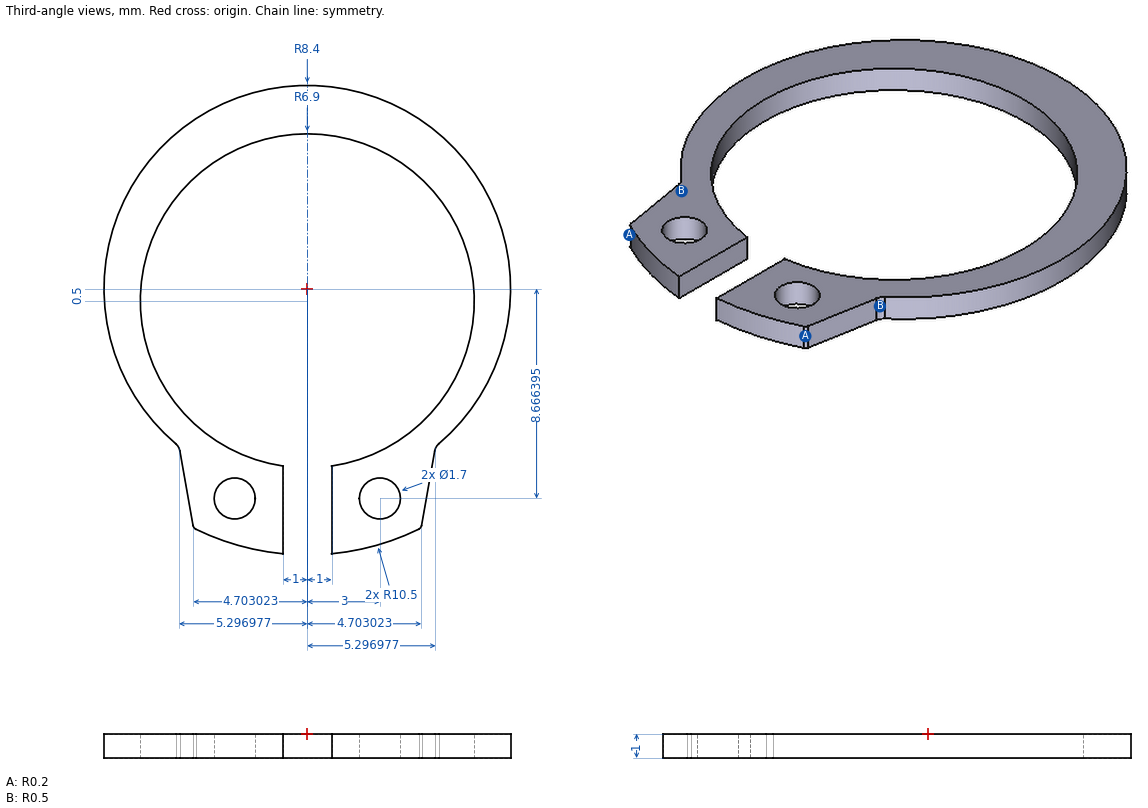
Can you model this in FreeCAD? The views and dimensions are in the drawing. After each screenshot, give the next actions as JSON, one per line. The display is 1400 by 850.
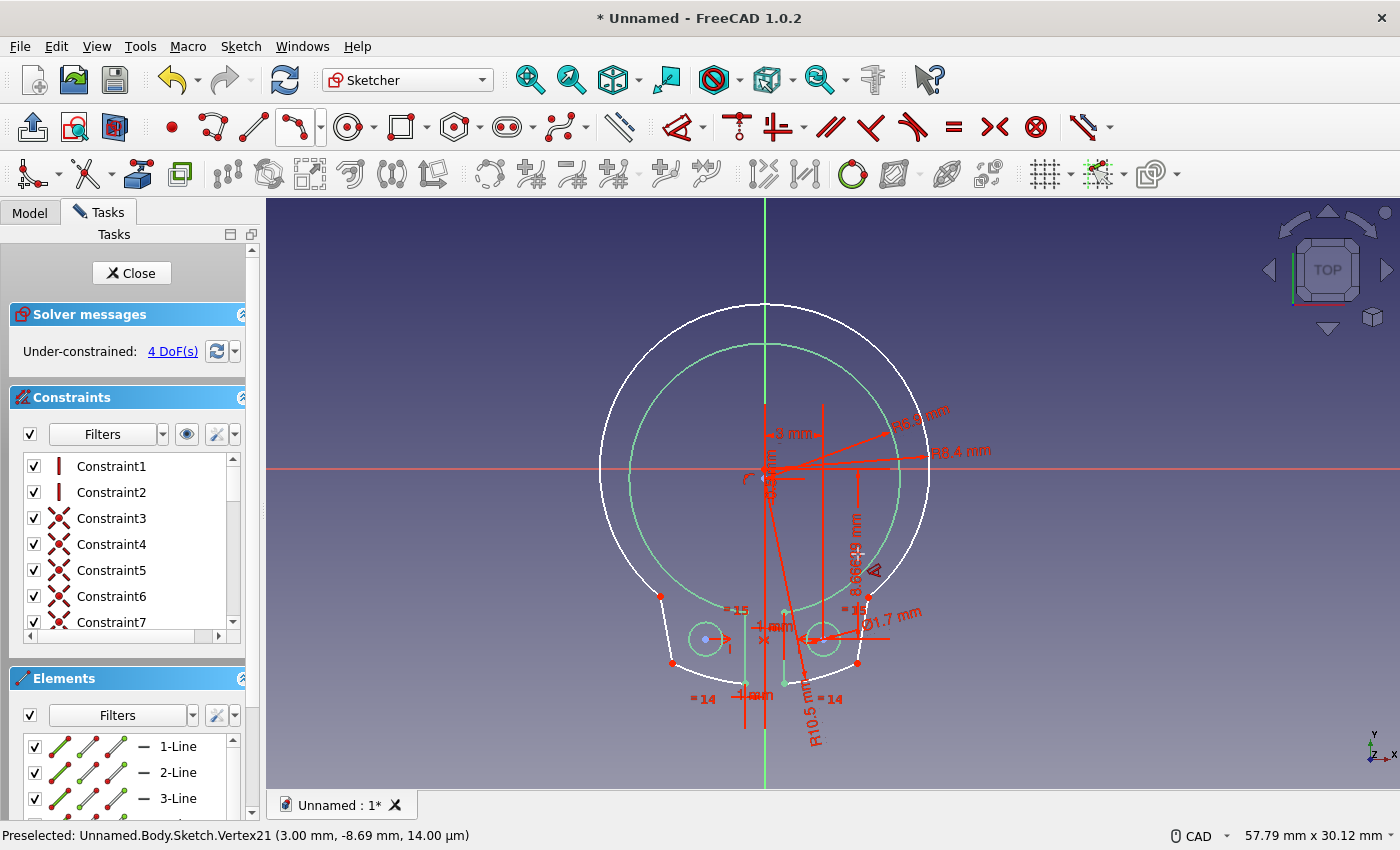
{"action": "left_click", "coordinate": [857, 663]}
{"action": "left_click", "coordinate": [811, 411]}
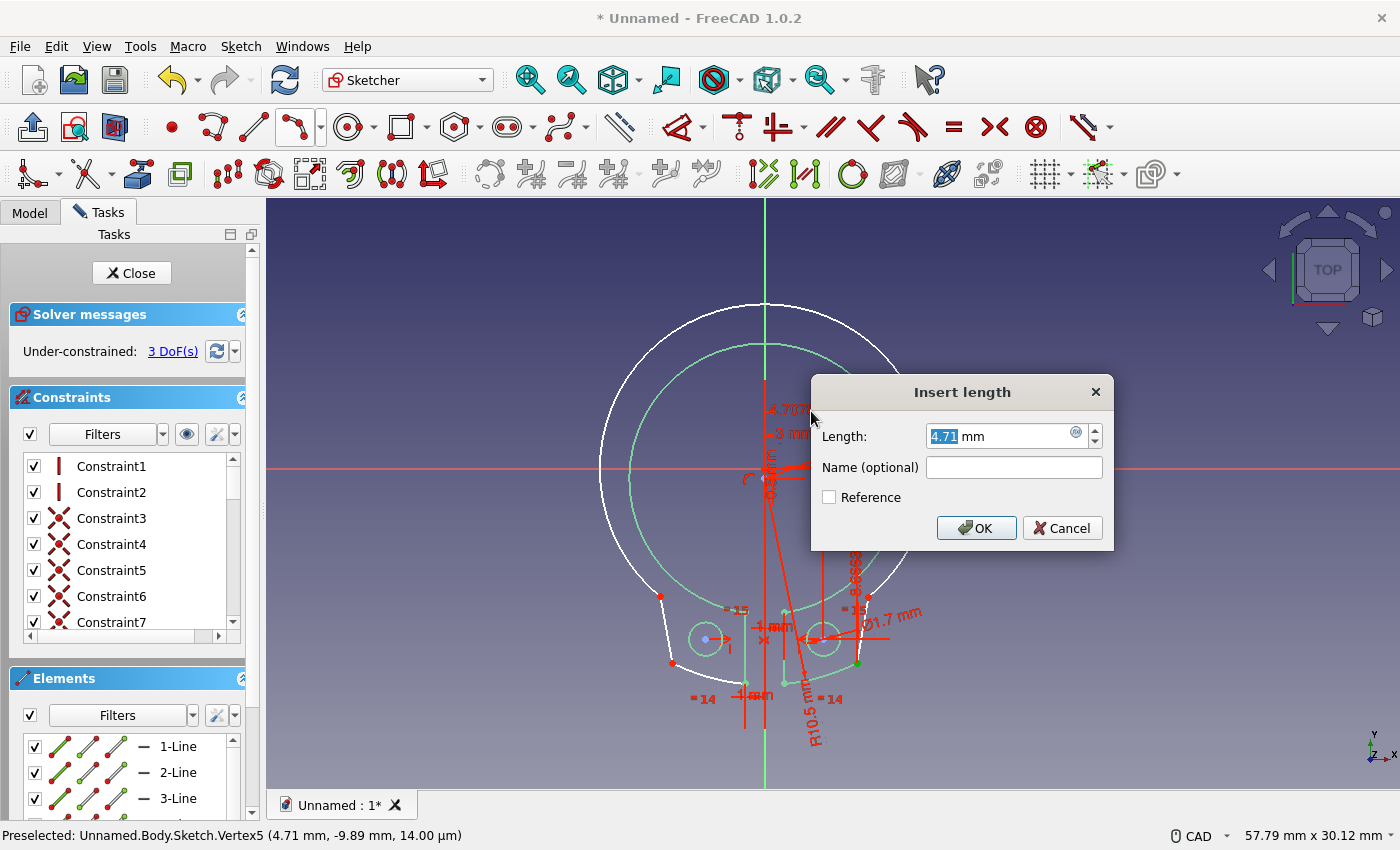
{"action": "type", "text": "4.703023"}
{"action": "key", "text": "Return"}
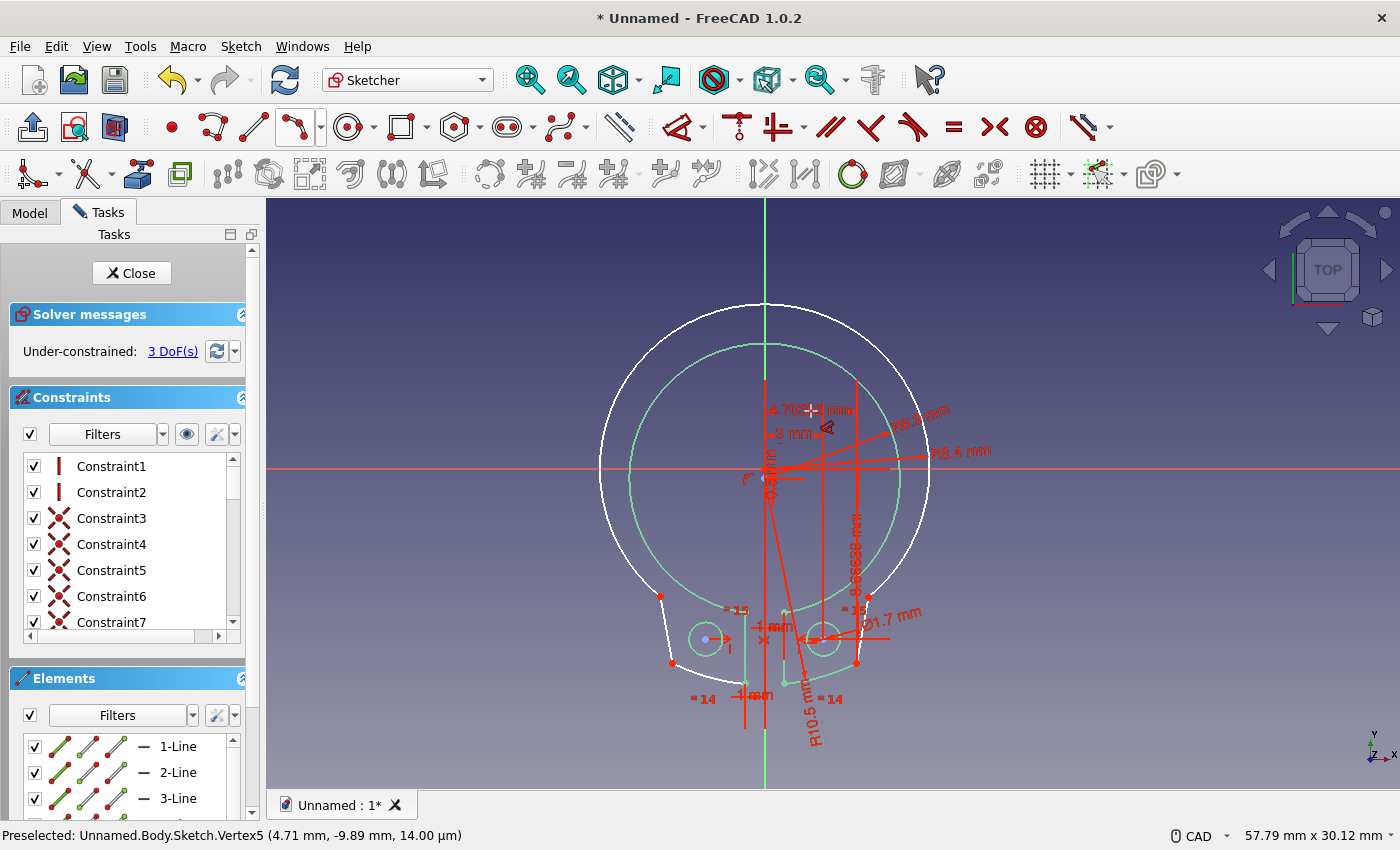
{"action": "left_click", "coordinate": [868, 597]}
{"action": "left_click", "coordinate": [817, 387]}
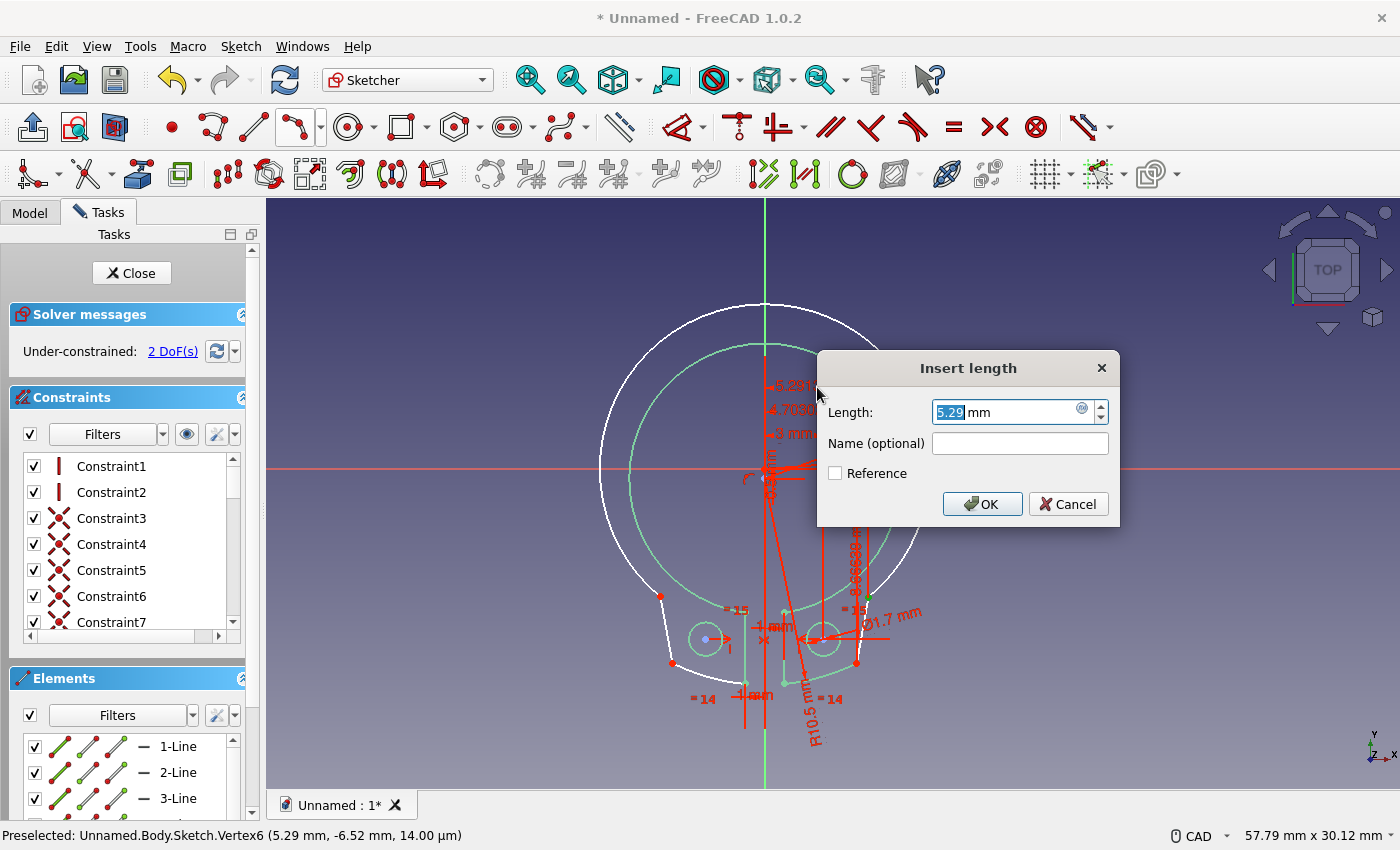
{"action": "type", "text": "5.296977"}
{"action": "key", "text": "Return"}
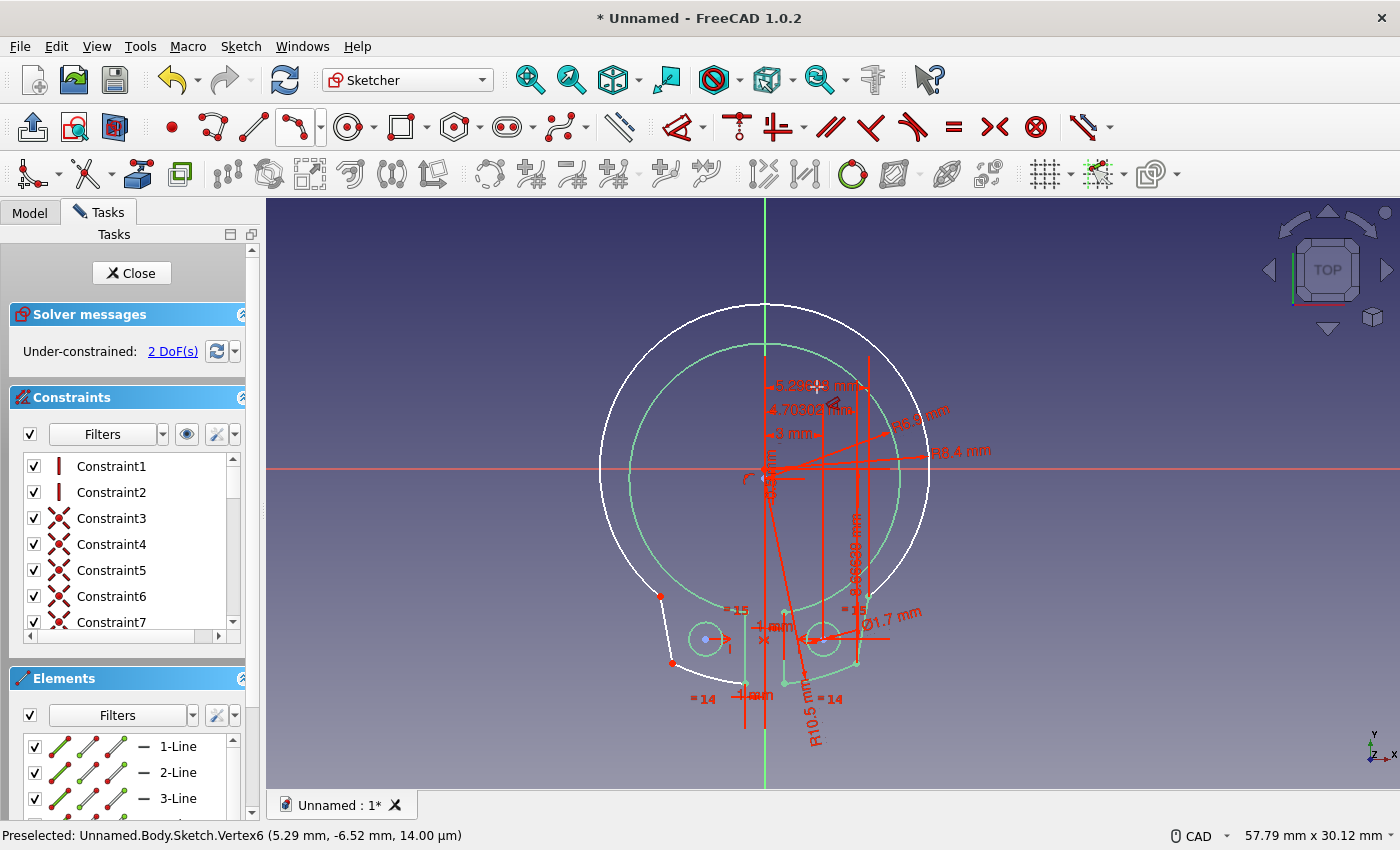
{"action": "left_click", "coordinate": [660, 597]}
{"action": "left_click", "coordinate": [713, 435]}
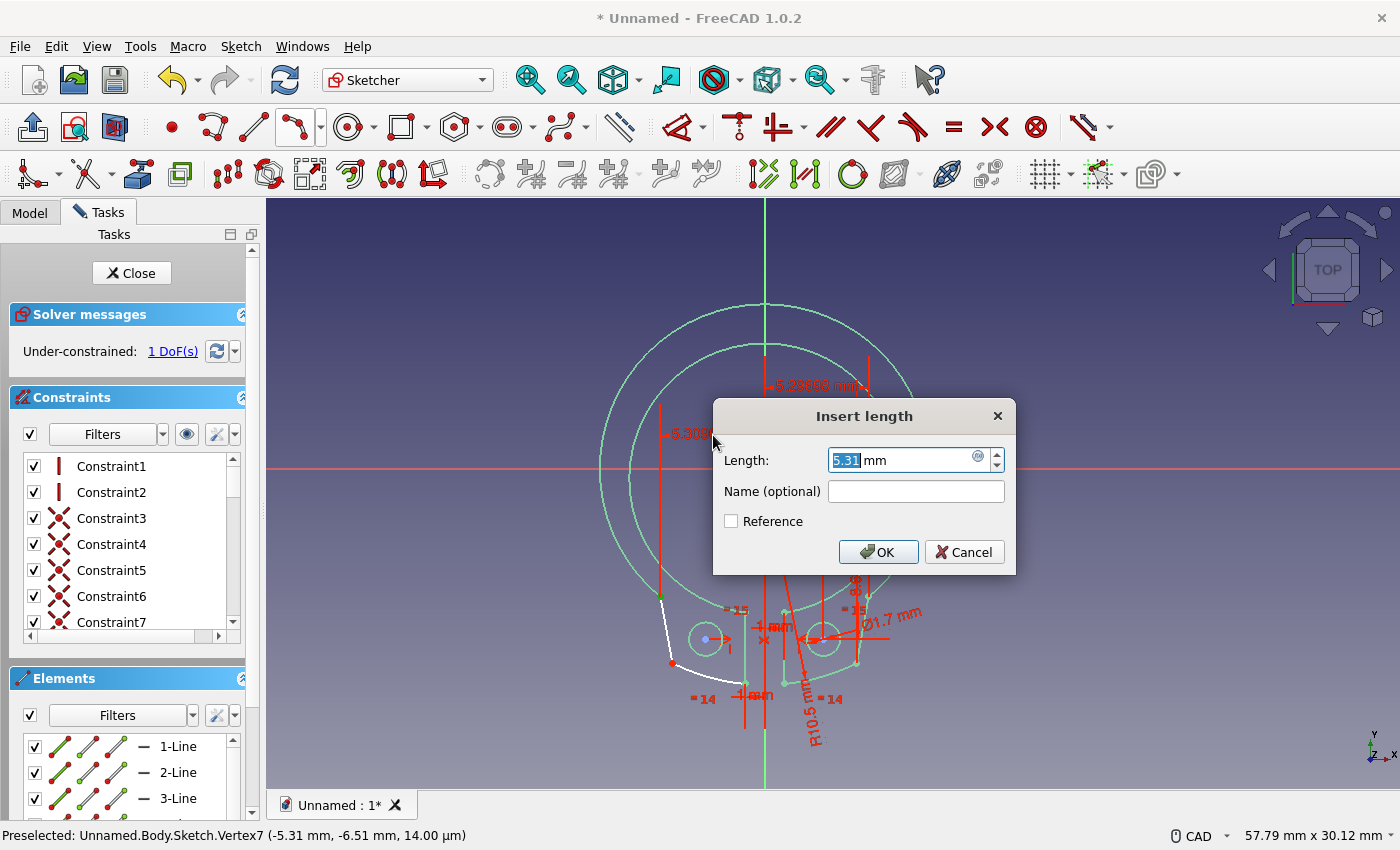
{"action": "type", "text": "5.296977"}
{"action": "key", "text": "Return"}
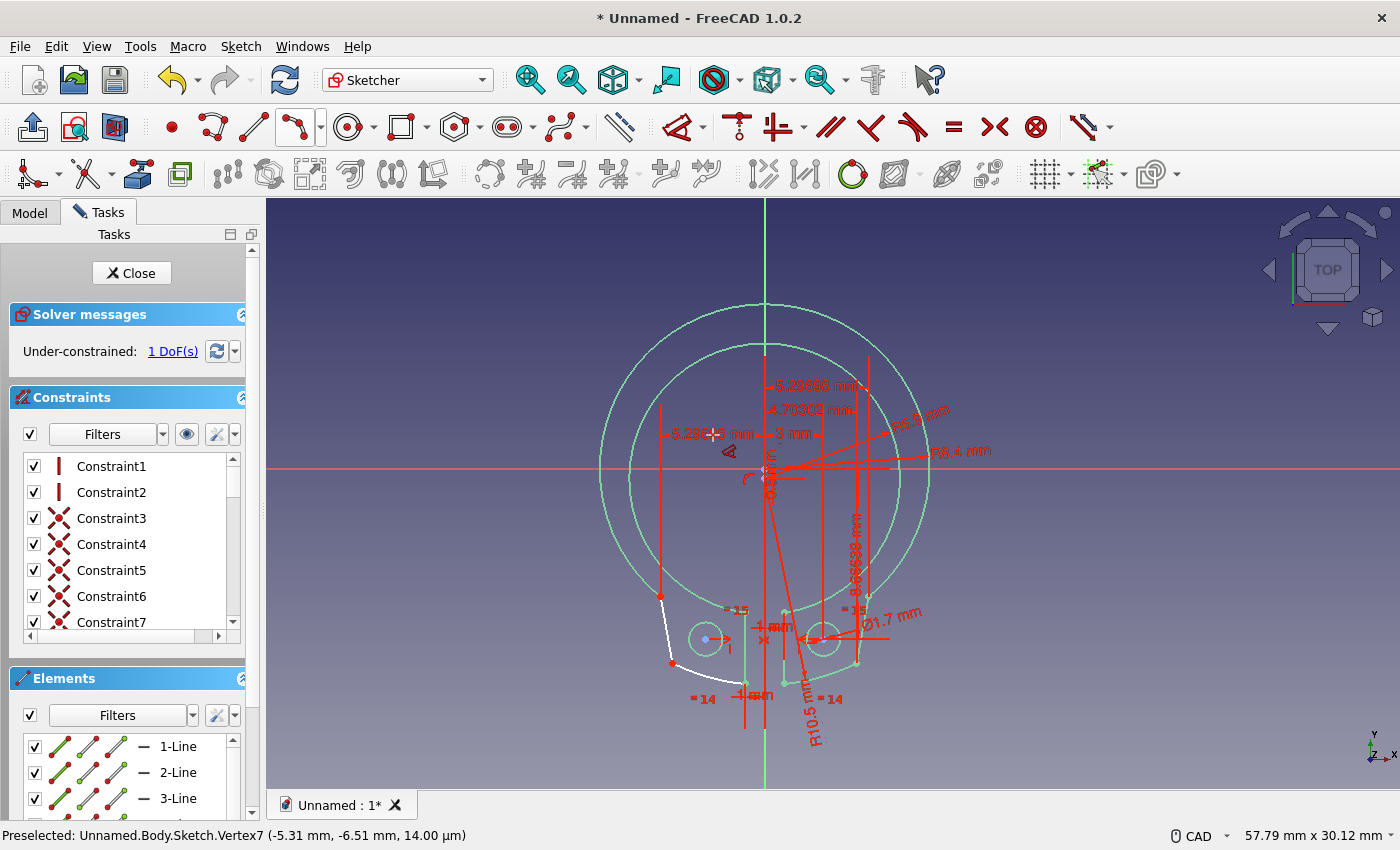
{"action": "left_click", "coordinate": [672, 663]}
{"action": "left_click", "coordinate": [719, 721]}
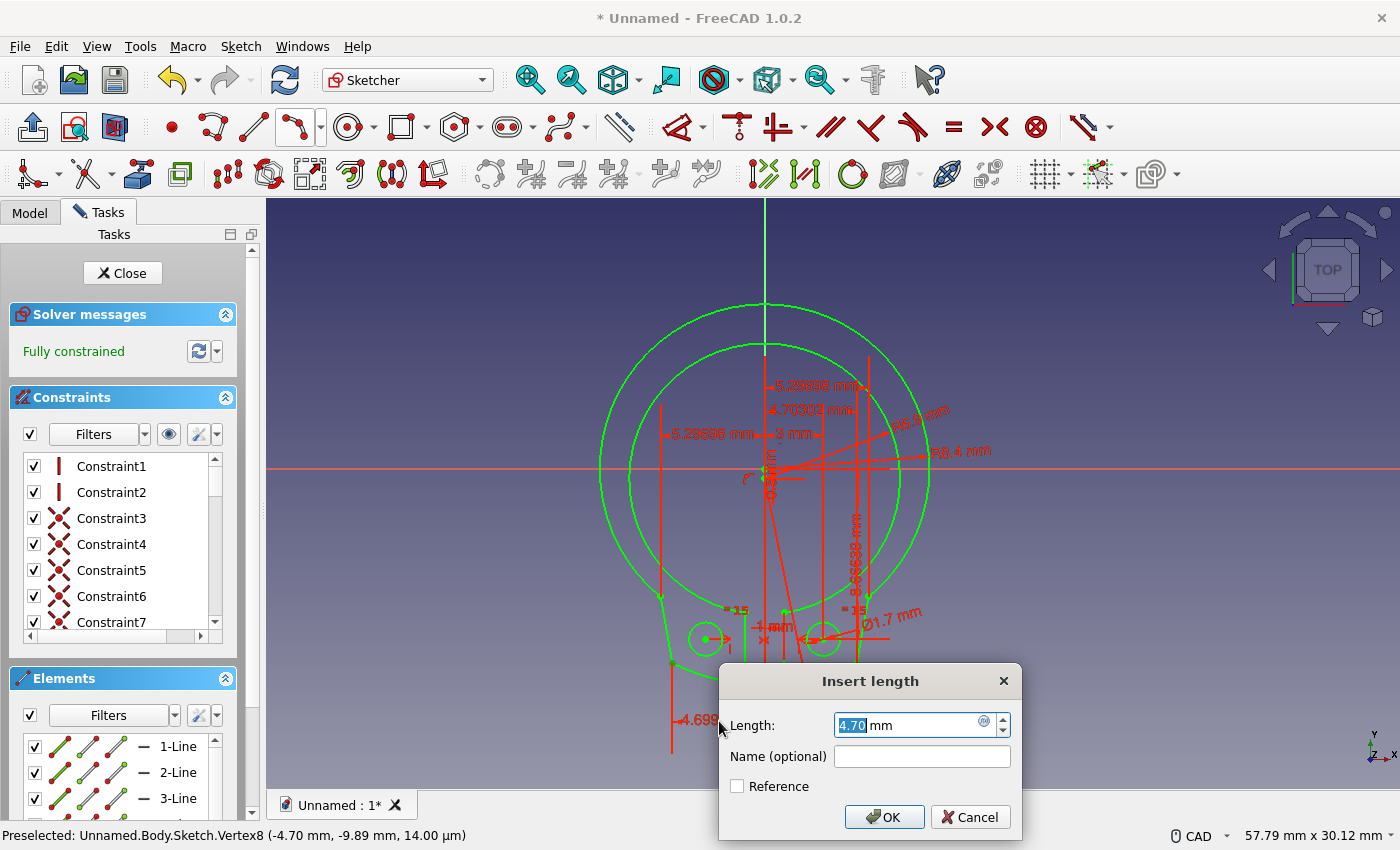
{"action": "type", "text": "4.703023"}
{"action": "key", "text": "Return"}
{"action": "key", "text": "Escape"}